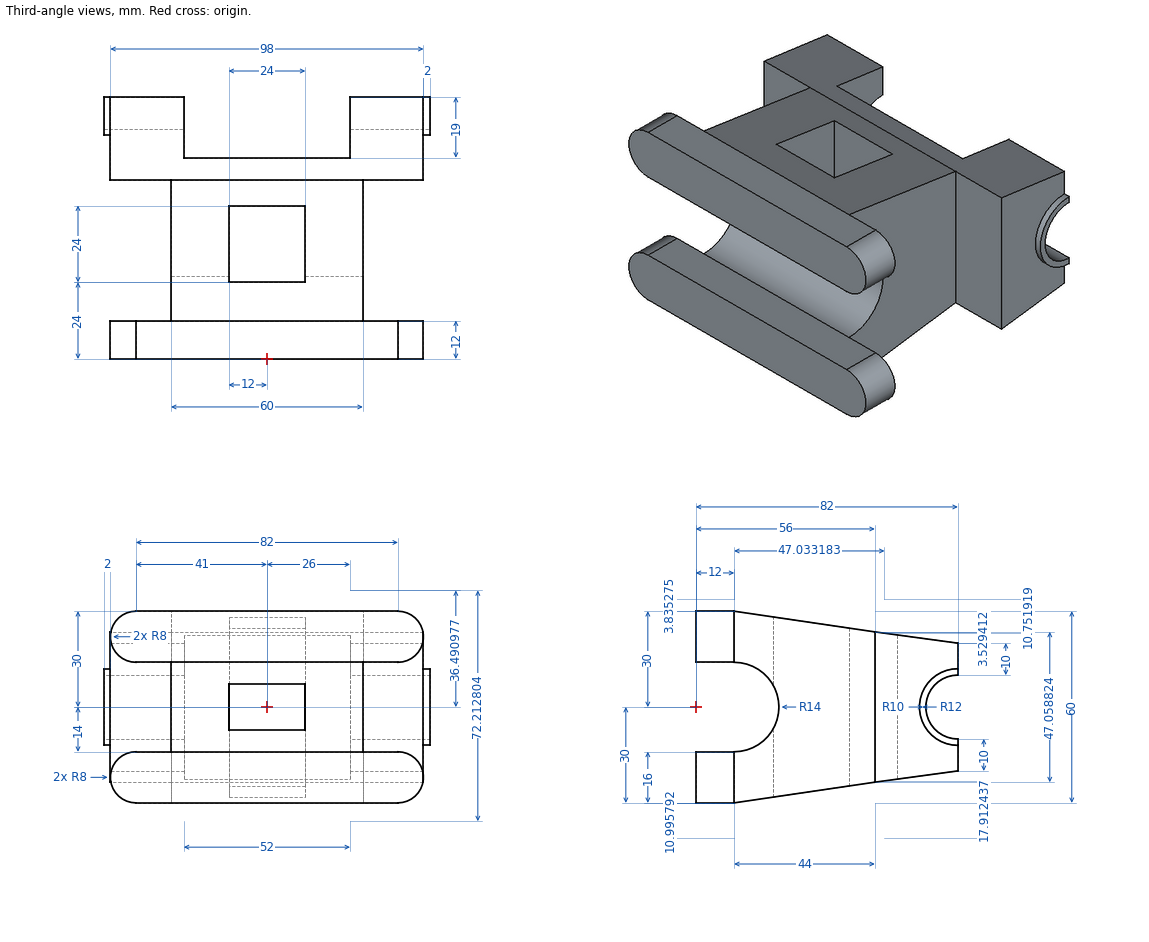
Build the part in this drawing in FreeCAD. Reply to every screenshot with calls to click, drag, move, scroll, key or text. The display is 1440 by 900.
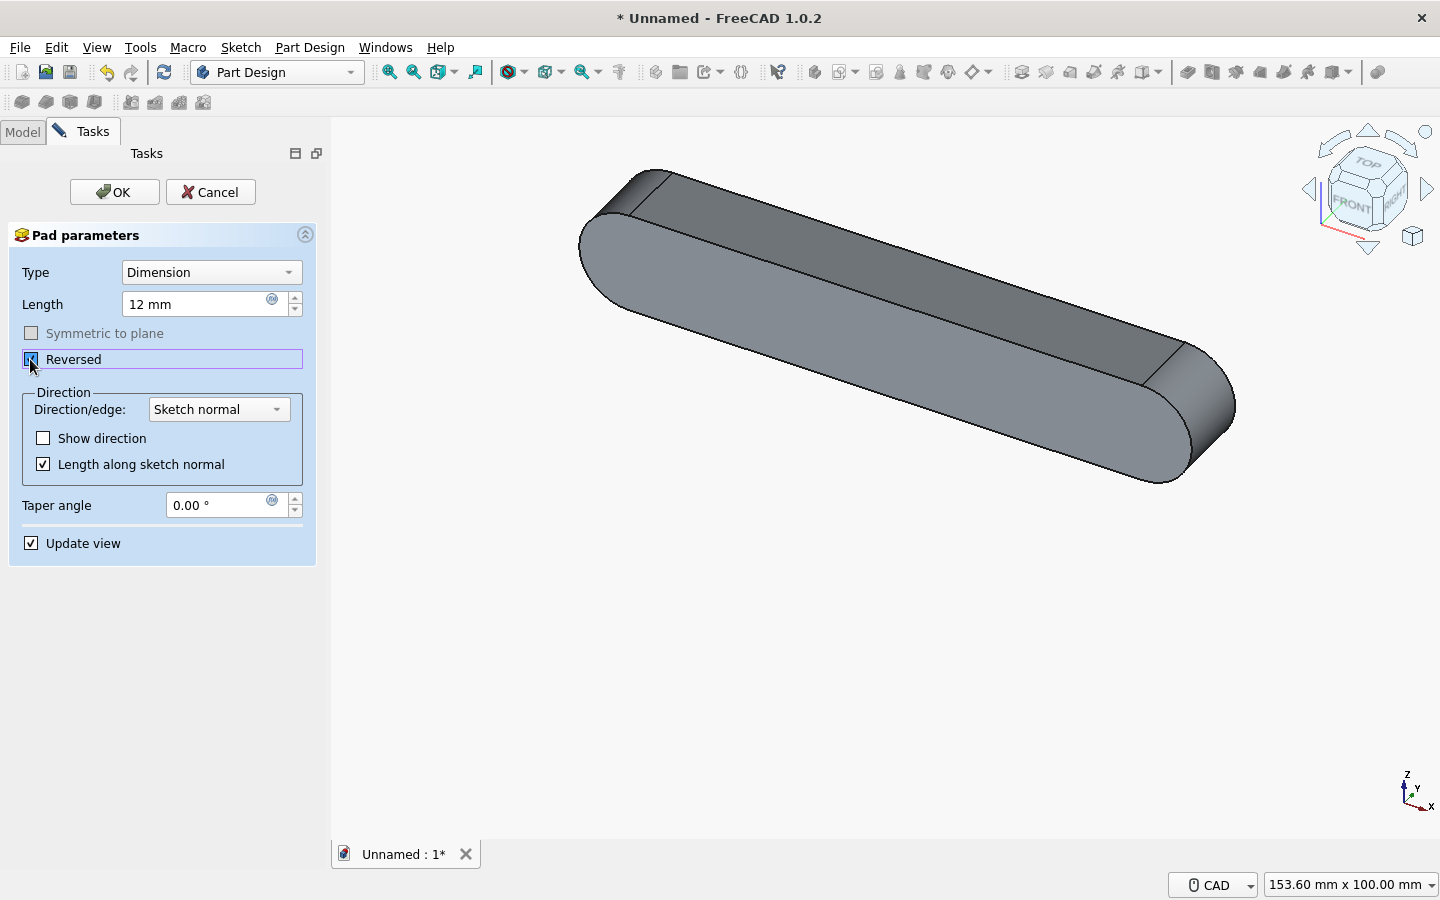
click(115, 192)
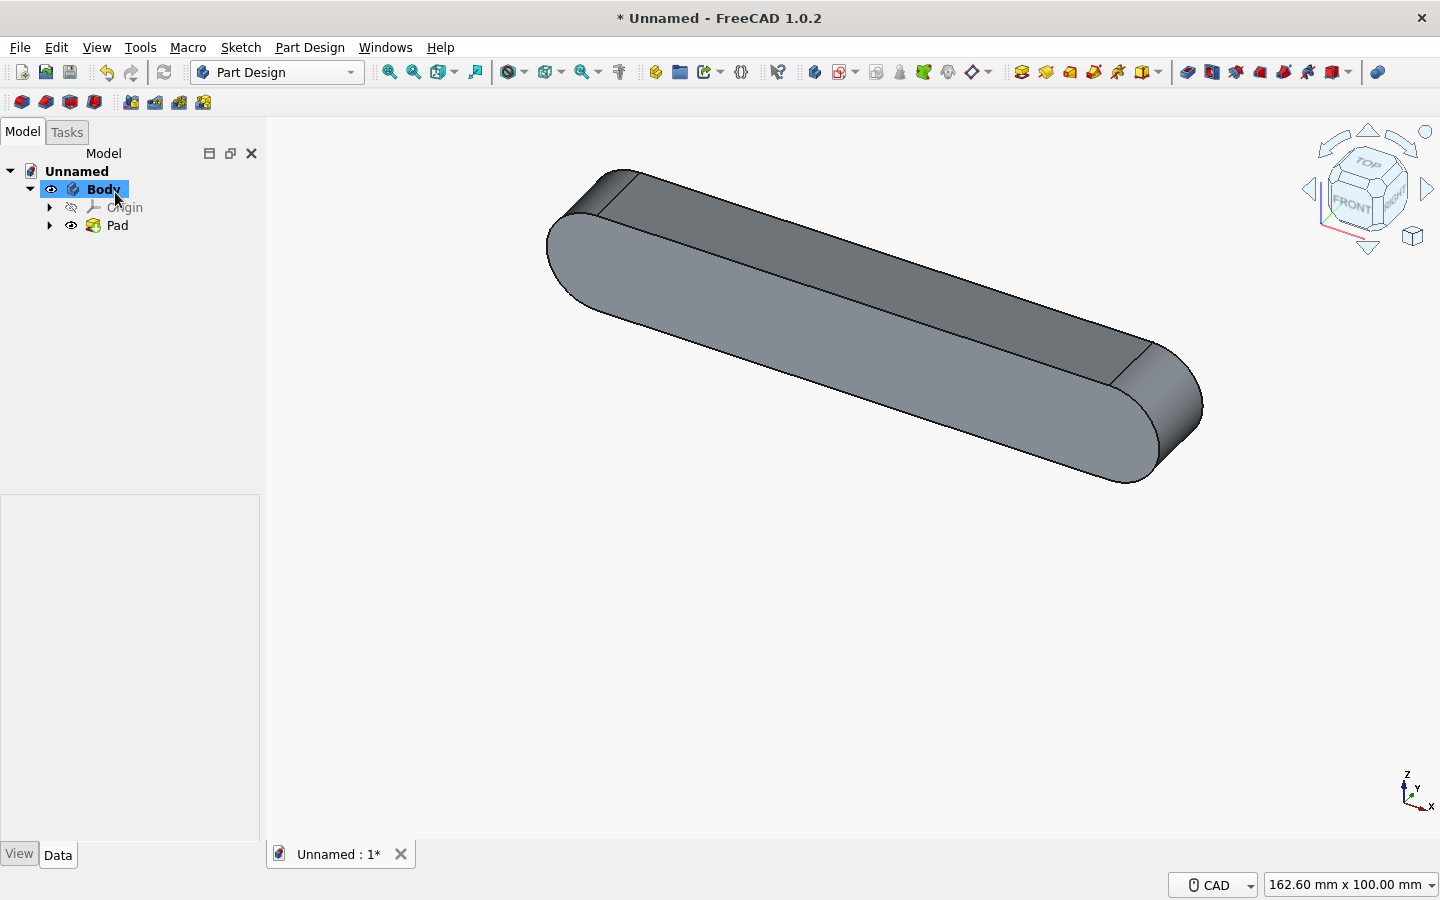
click(816, 72)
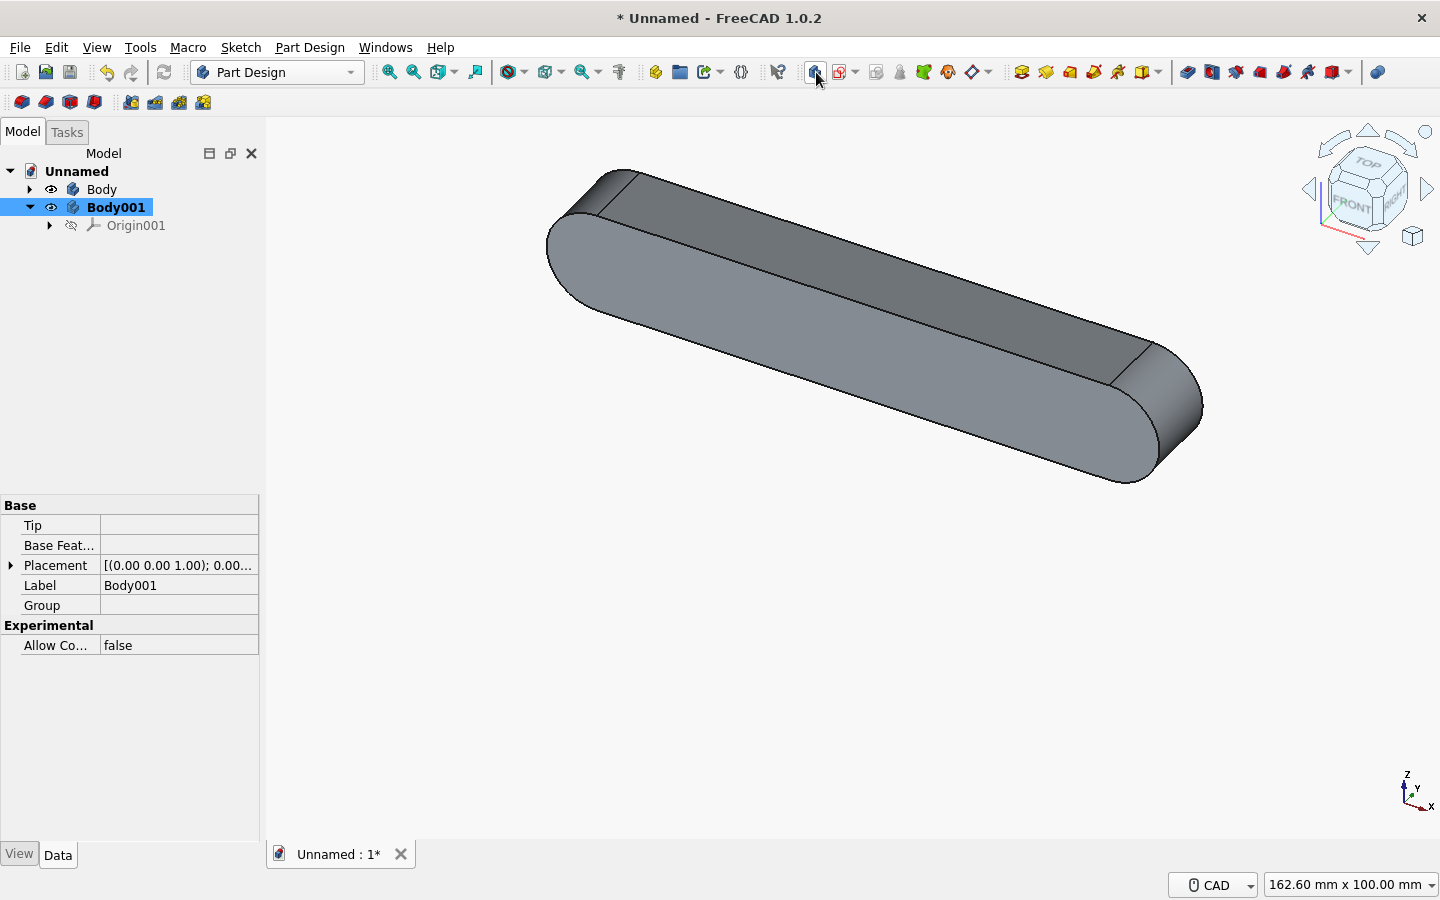
click(306, 799)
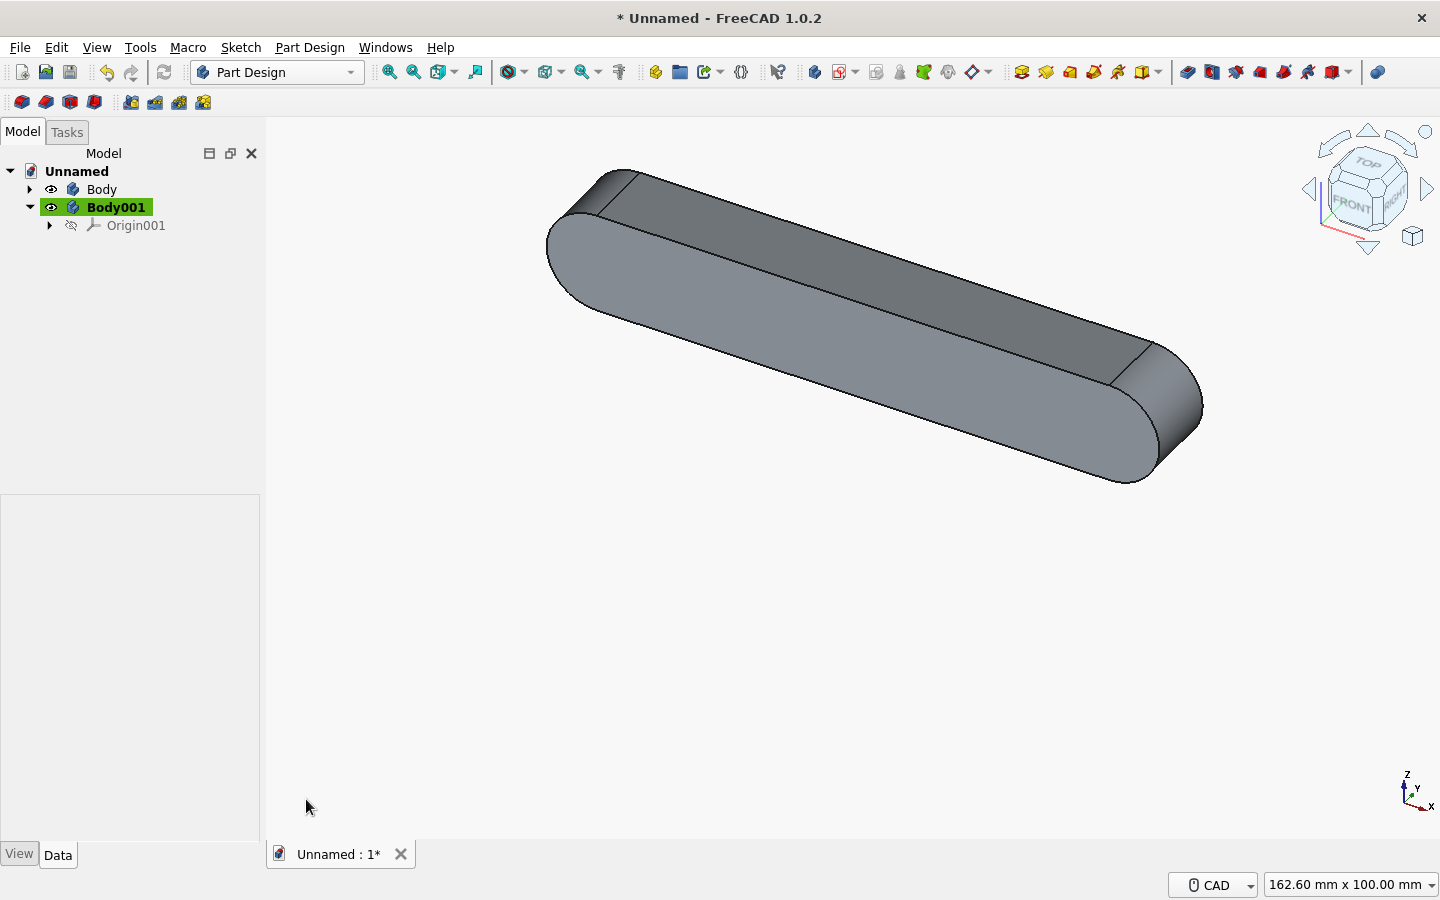
click(840, 72)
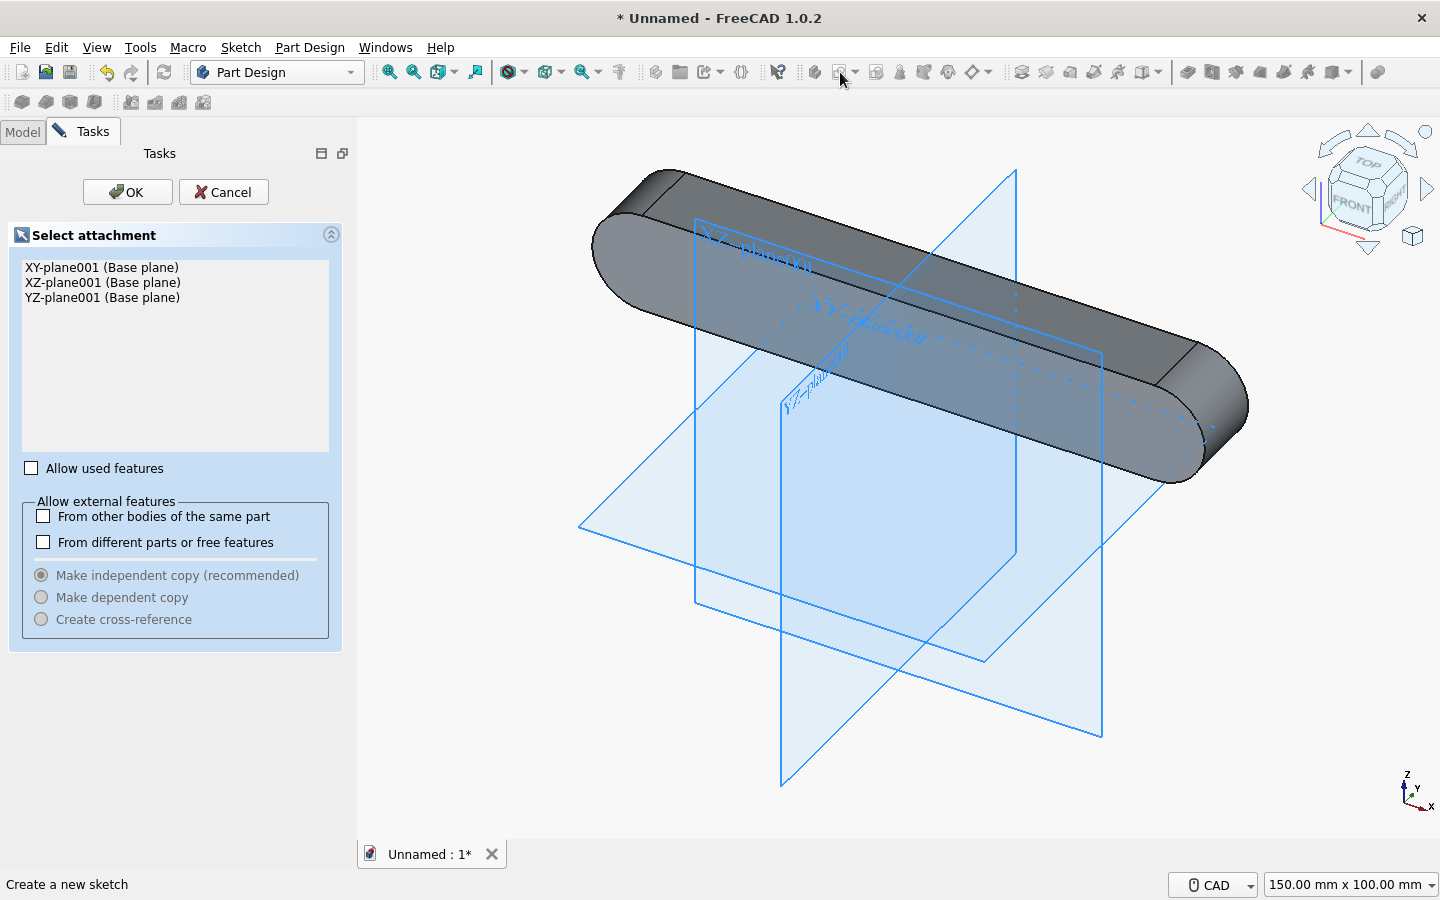
click(82, 282)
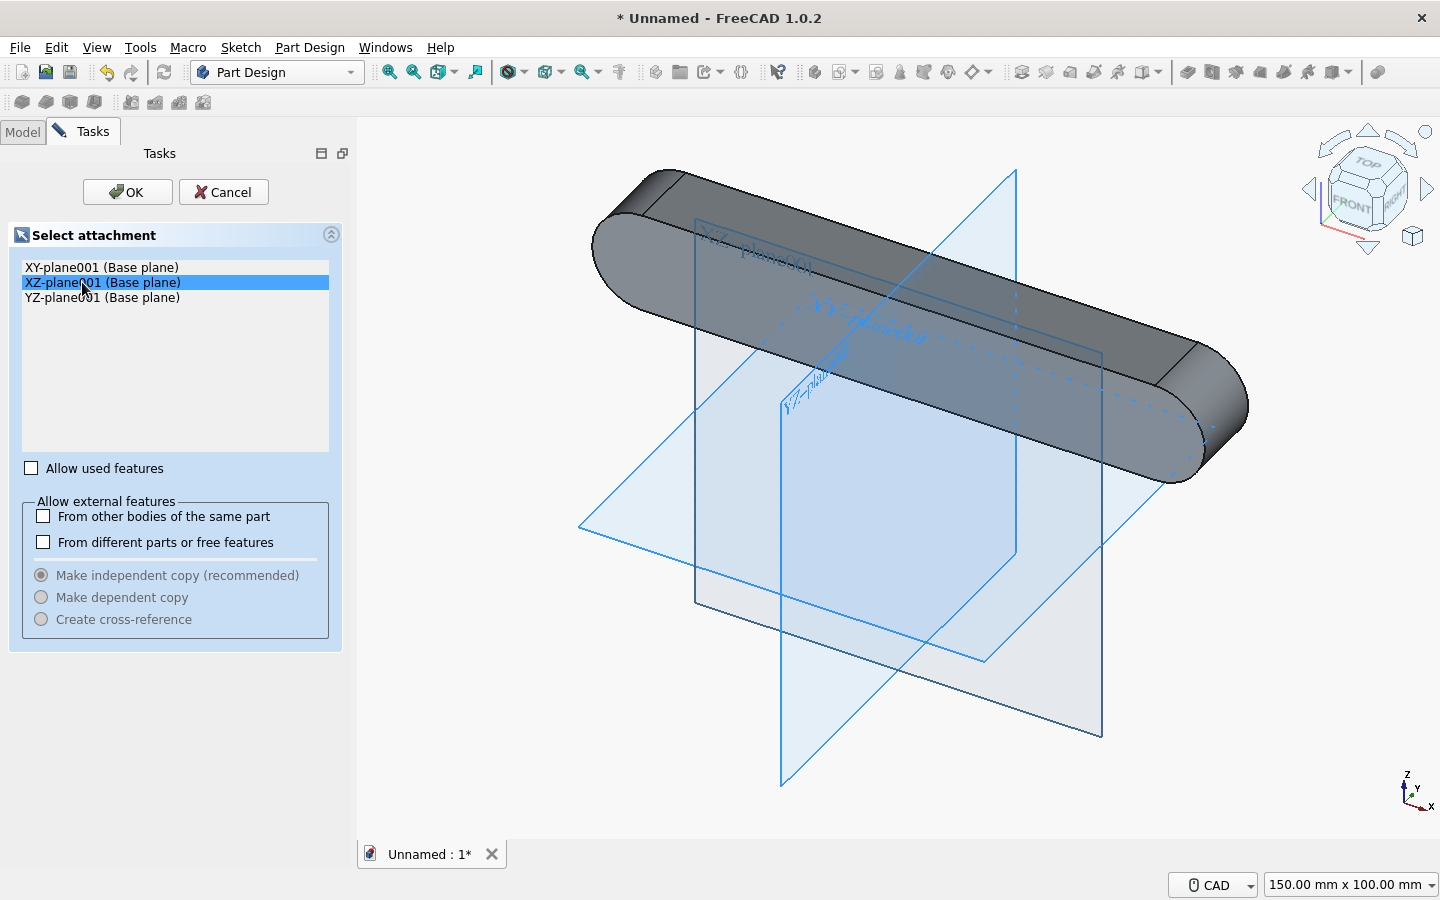
click(128, 192)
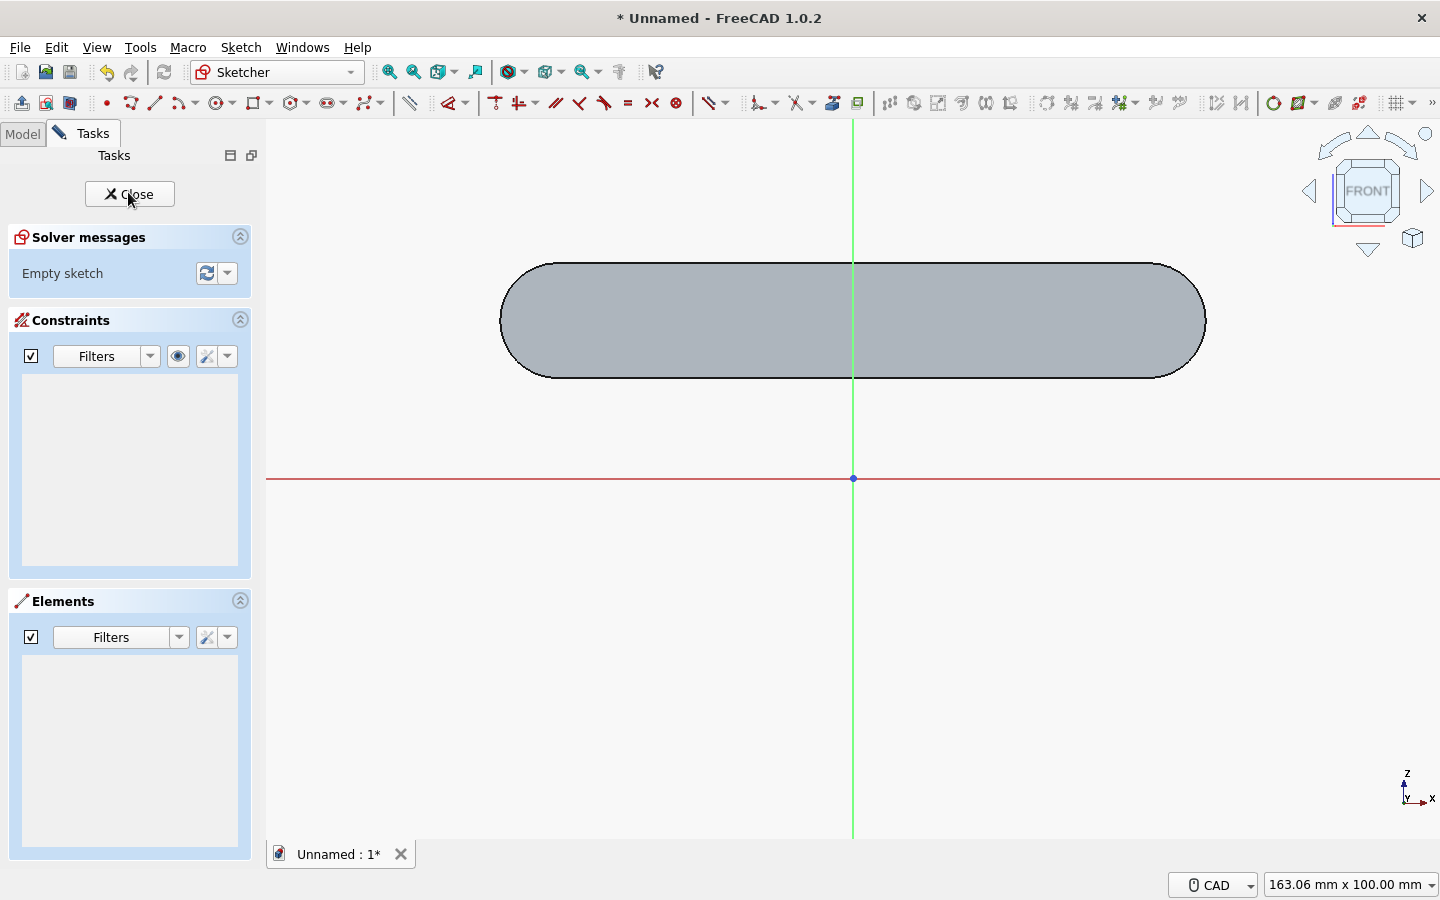
click(328, 104)